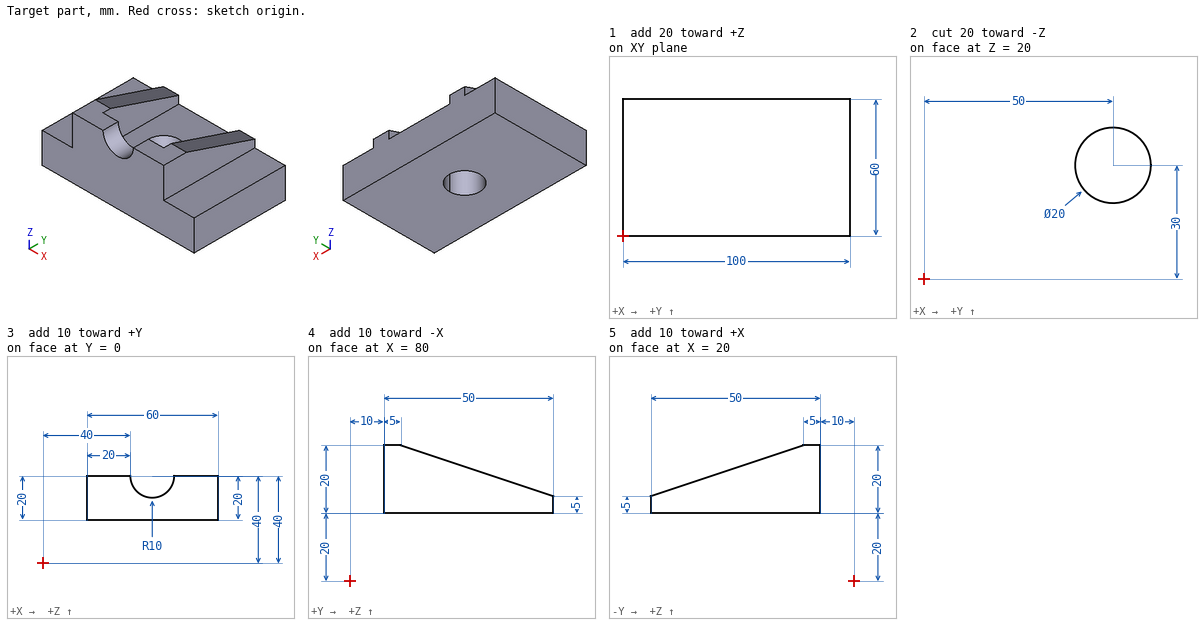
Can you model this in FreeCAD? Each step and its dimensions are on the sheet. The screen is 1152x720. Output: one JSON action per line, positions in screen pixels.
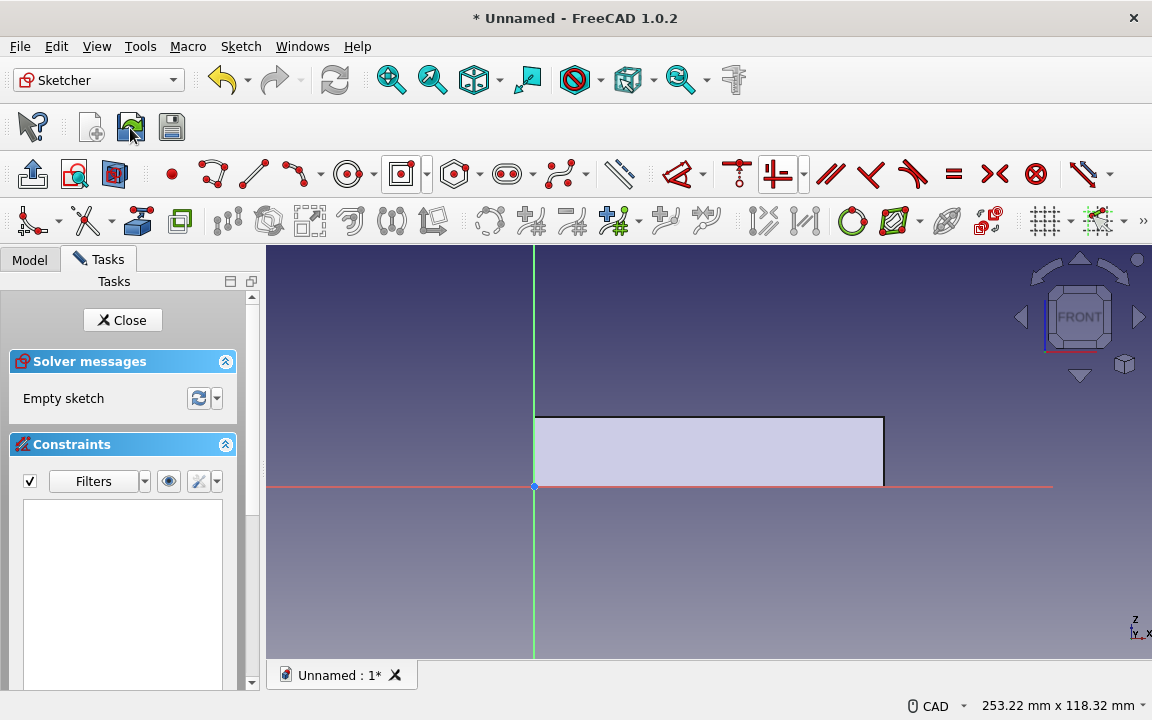
{"action": "scroll", "coordinate": [715, 374], "scroll_direction": "up", "scroll_amount": 3}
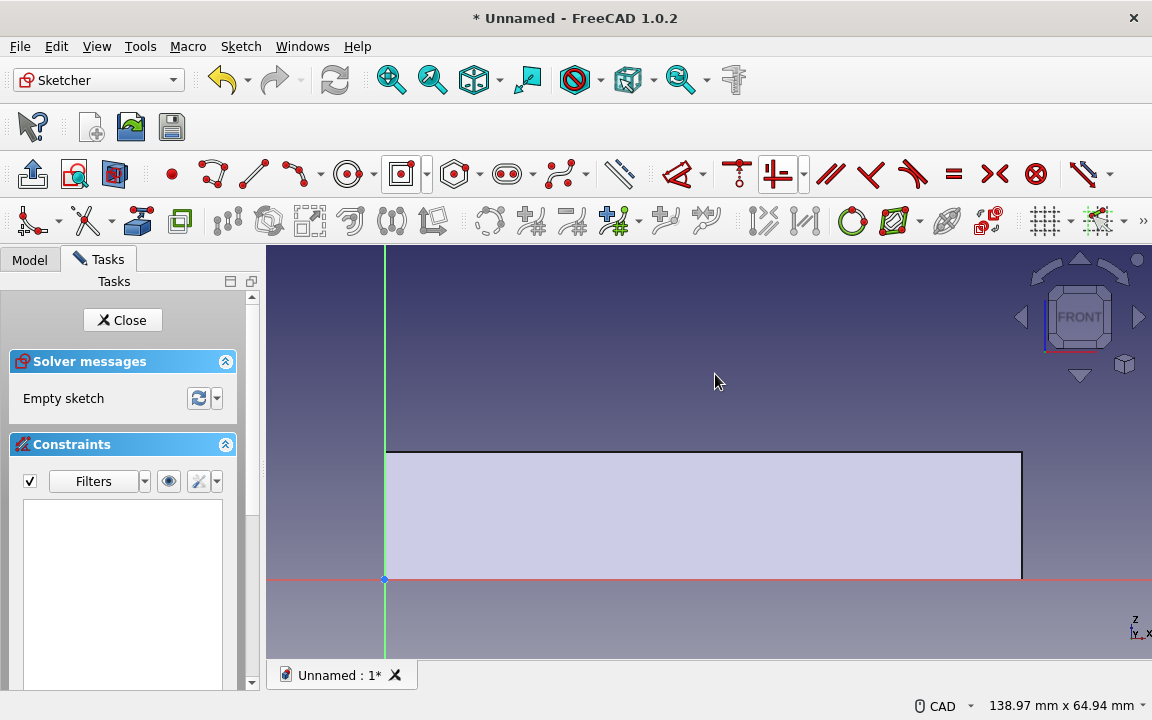
{"action": "left_click", "coordinate": [213, 174]}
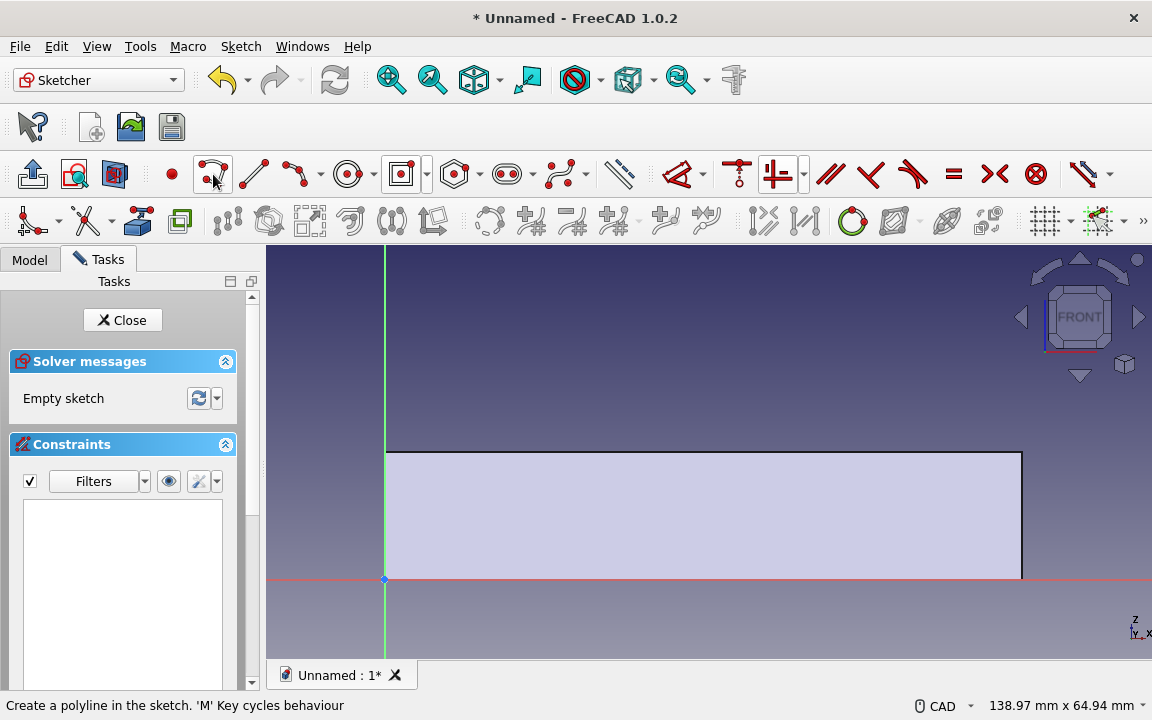
{"action": "left_click", "coordinate": [640, 325]}
{"action": "left_click", "coordinate": [512, 325]}
{"action": "left_click", "coordinate": [512, 452]}
{"action": "left_click", "coordinate": [895, 452]}
{"action": "left_click", "coordinate": [895, 325]}
{"action": "left_click", "coordinate": [767, 325]}
{"action": "right_click", "coordinate": [767, 325]}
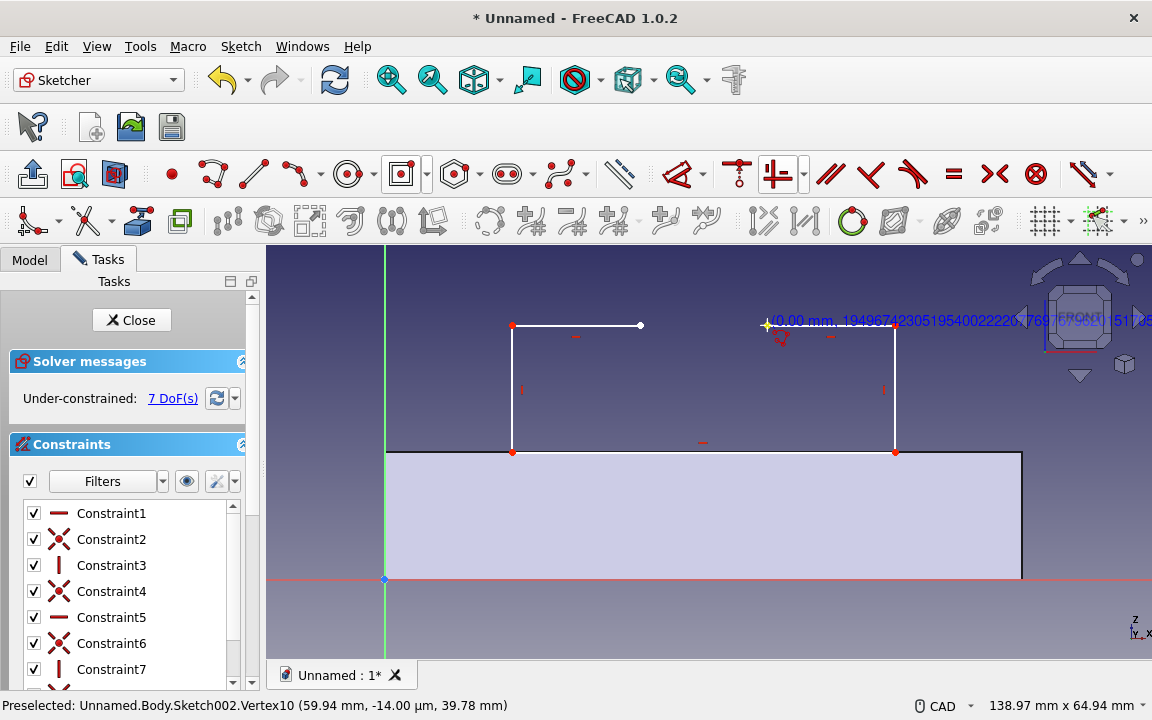
{"action": "left_click", "coordinate": [294, 174]}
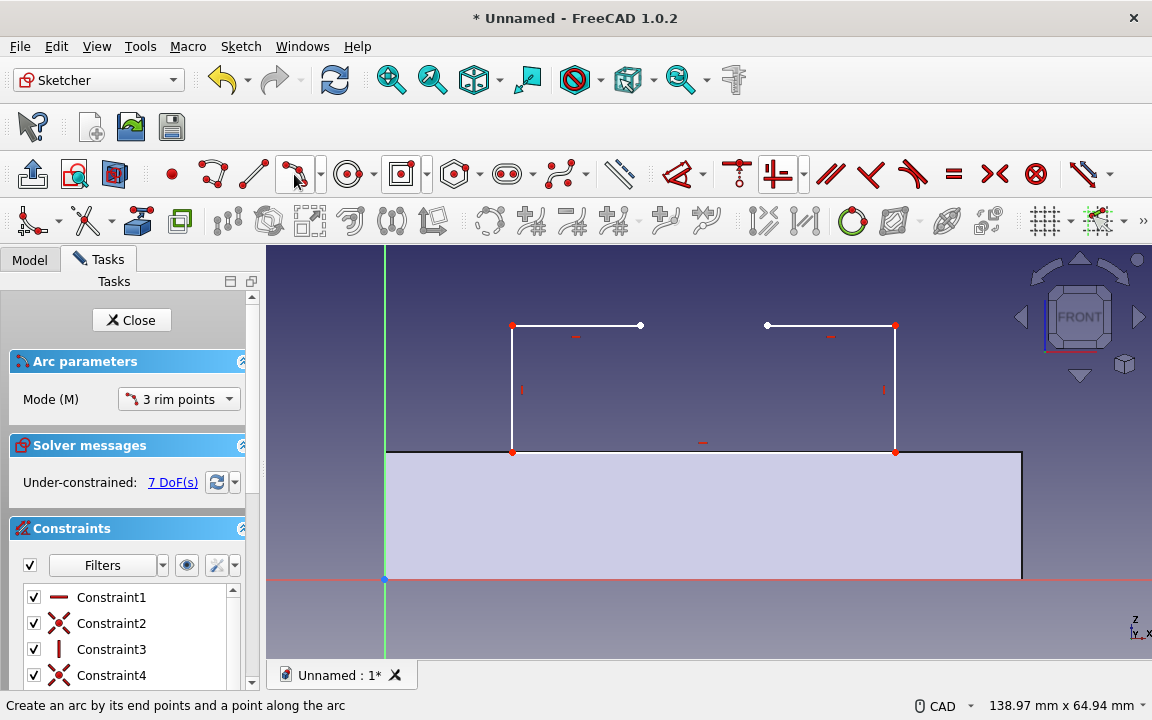
{"action": "left_click", "coordinate": [767, 326]}
{"action": "left_click", "coordinate": [640, 326]}
{"action": "left_click", "coordinate": [704, 388]}
{"action": "key", "text": "Escape"}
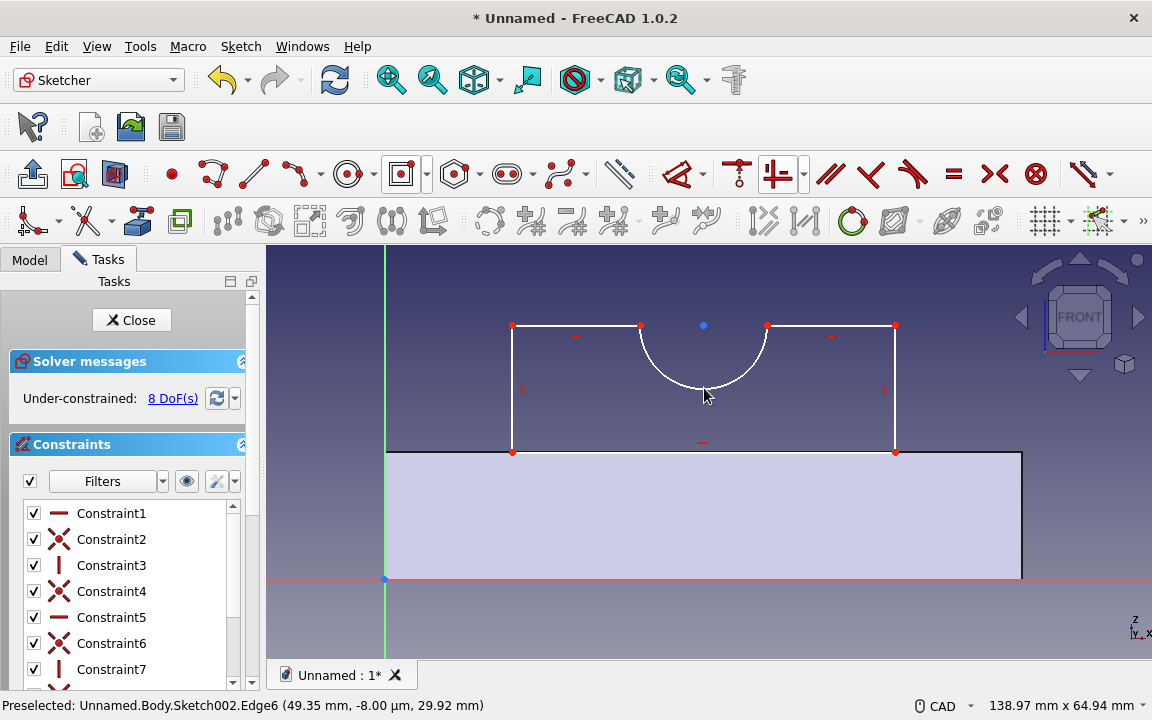
{"action": "left_click", "coordinate": [676, 174]}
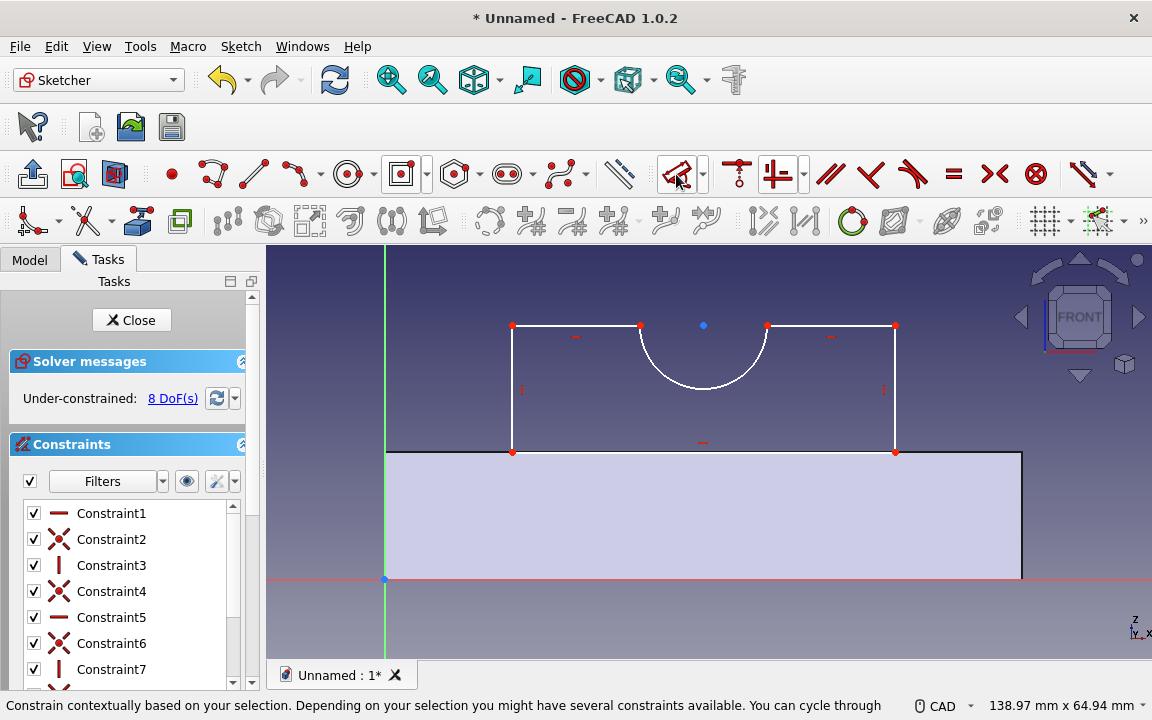
{"action": "left_click", "coordinate": [666, 377]}
{"action": "left_click", "coordinate": [647, 403]}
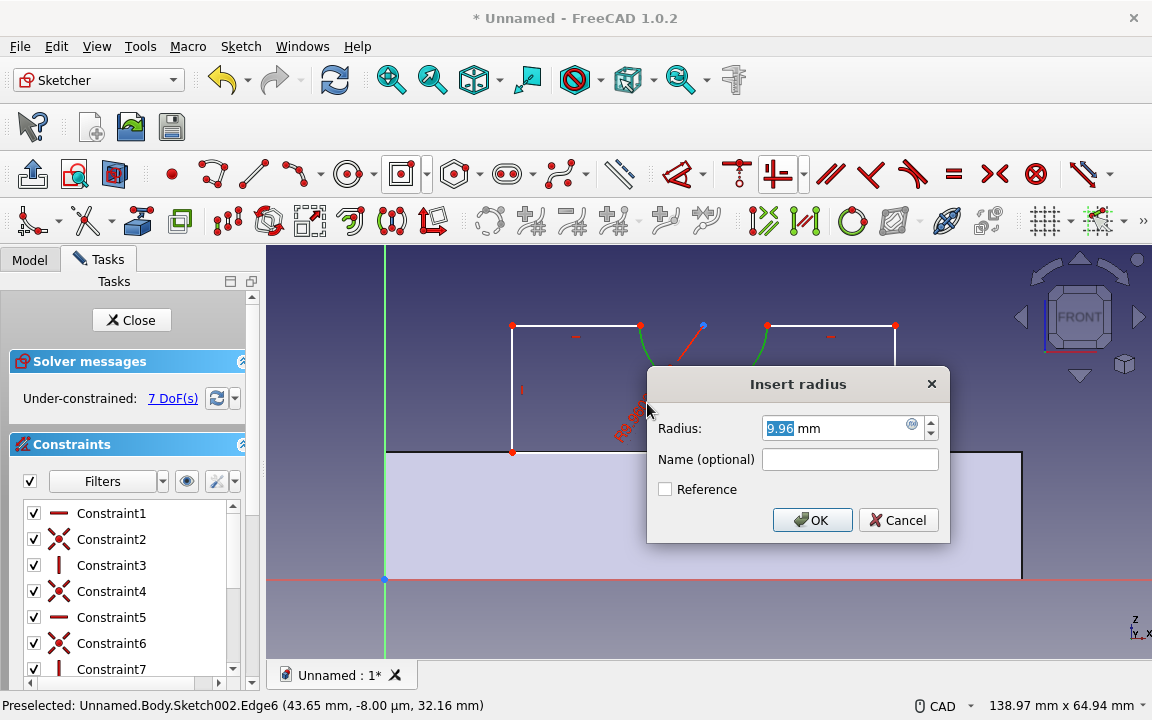
{"action": "type", "text": "10"}
{"action": "key", "text": "Return"}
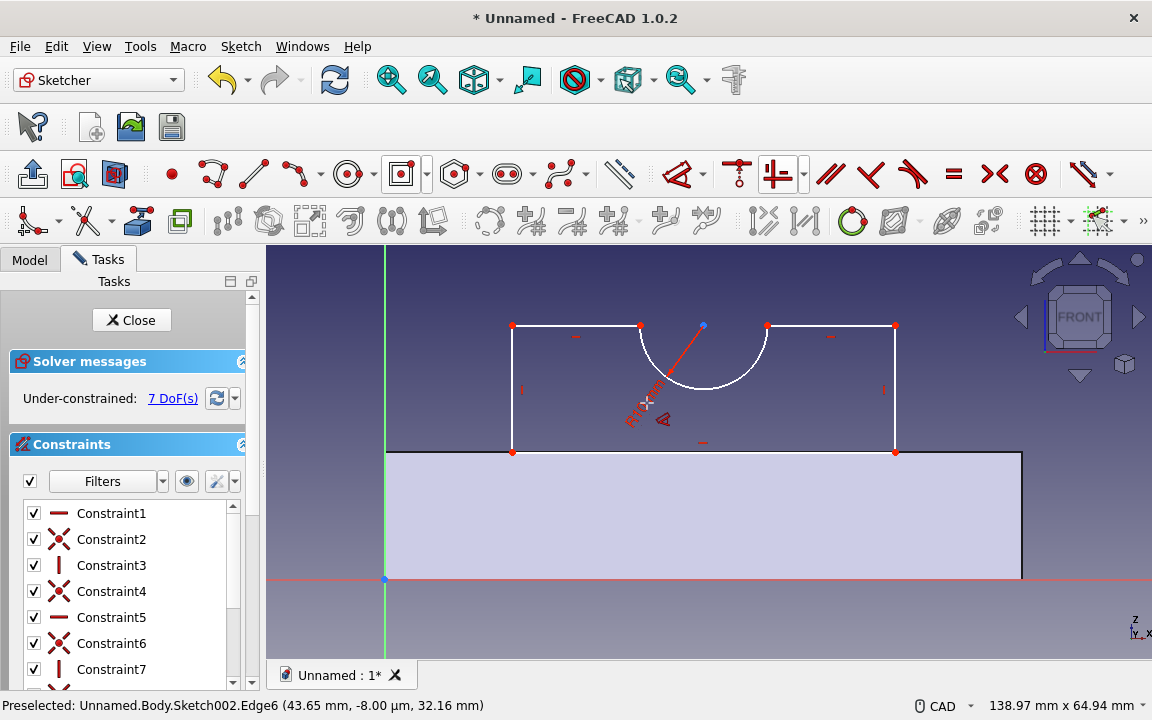
{"action": "left_click", "coordinate": [602, 326]}
{"action": "left_click", "coordinate": [576, 292]}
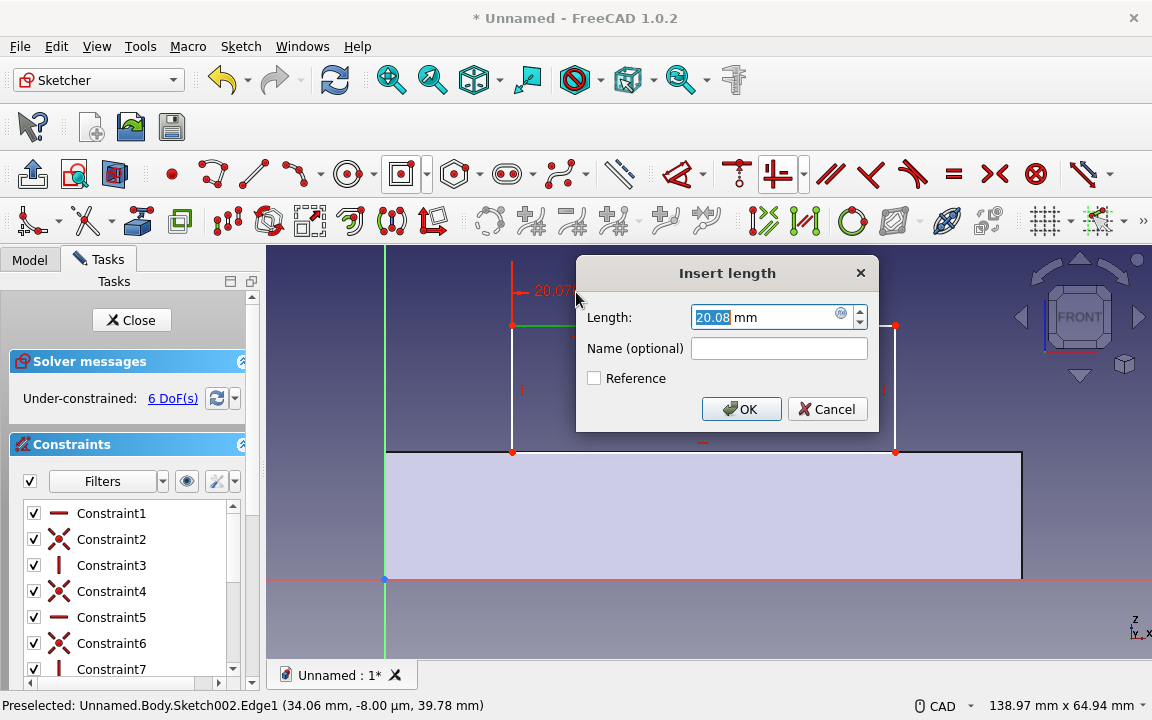
{"action": "type", "text": "20"}
{"action": "key", "text": "Return"}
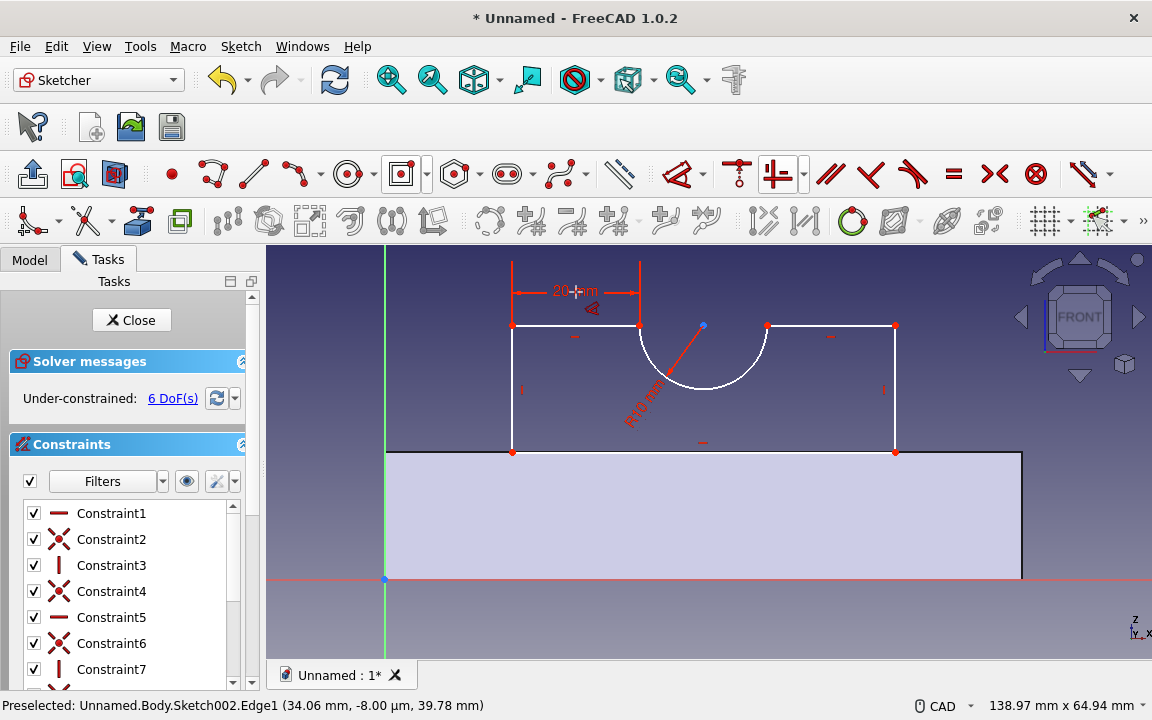
{"action": "left_click", "coordinate": [512, 364]}
{"action": "left_click", "coordinate": [478, 390]}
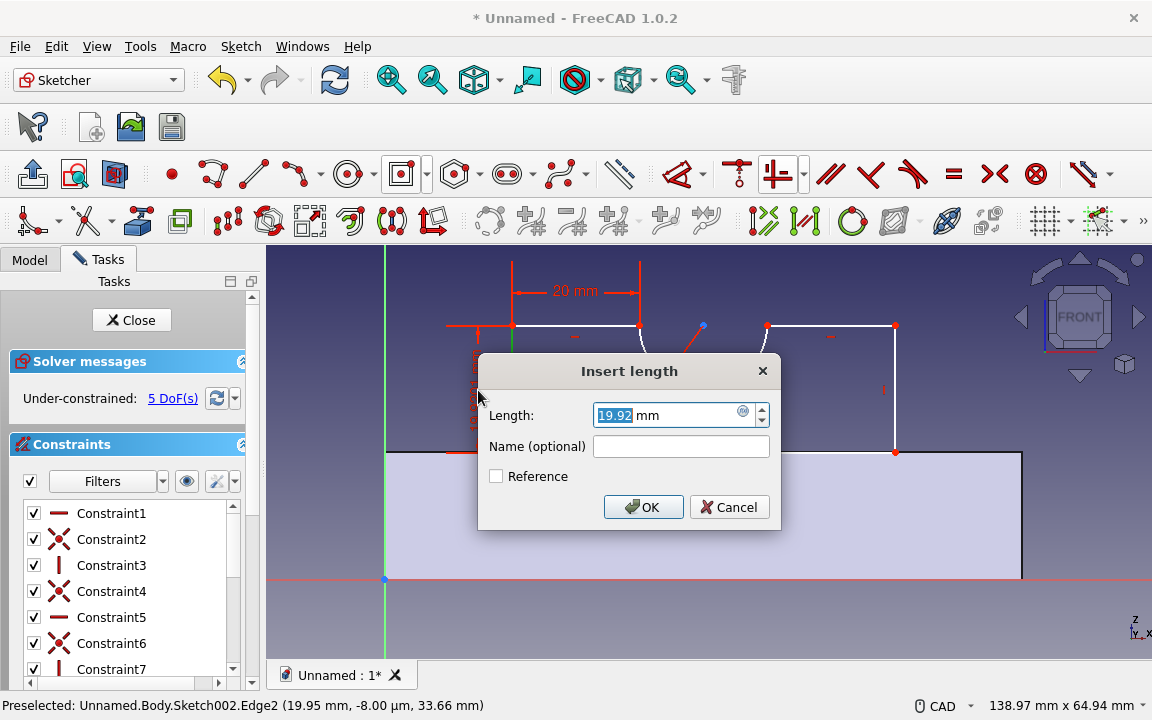
{"action": "type", "text": "20"}
{"action": "key", "text": "Return"}